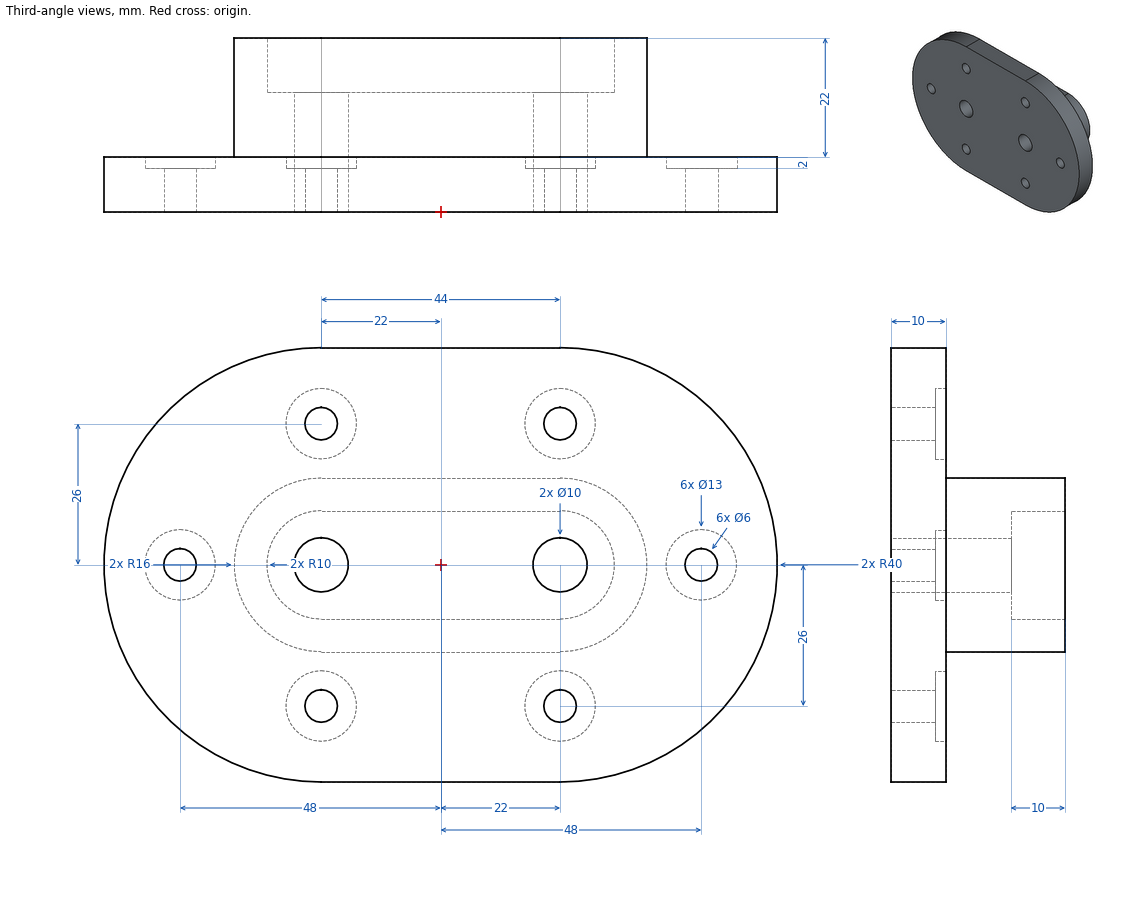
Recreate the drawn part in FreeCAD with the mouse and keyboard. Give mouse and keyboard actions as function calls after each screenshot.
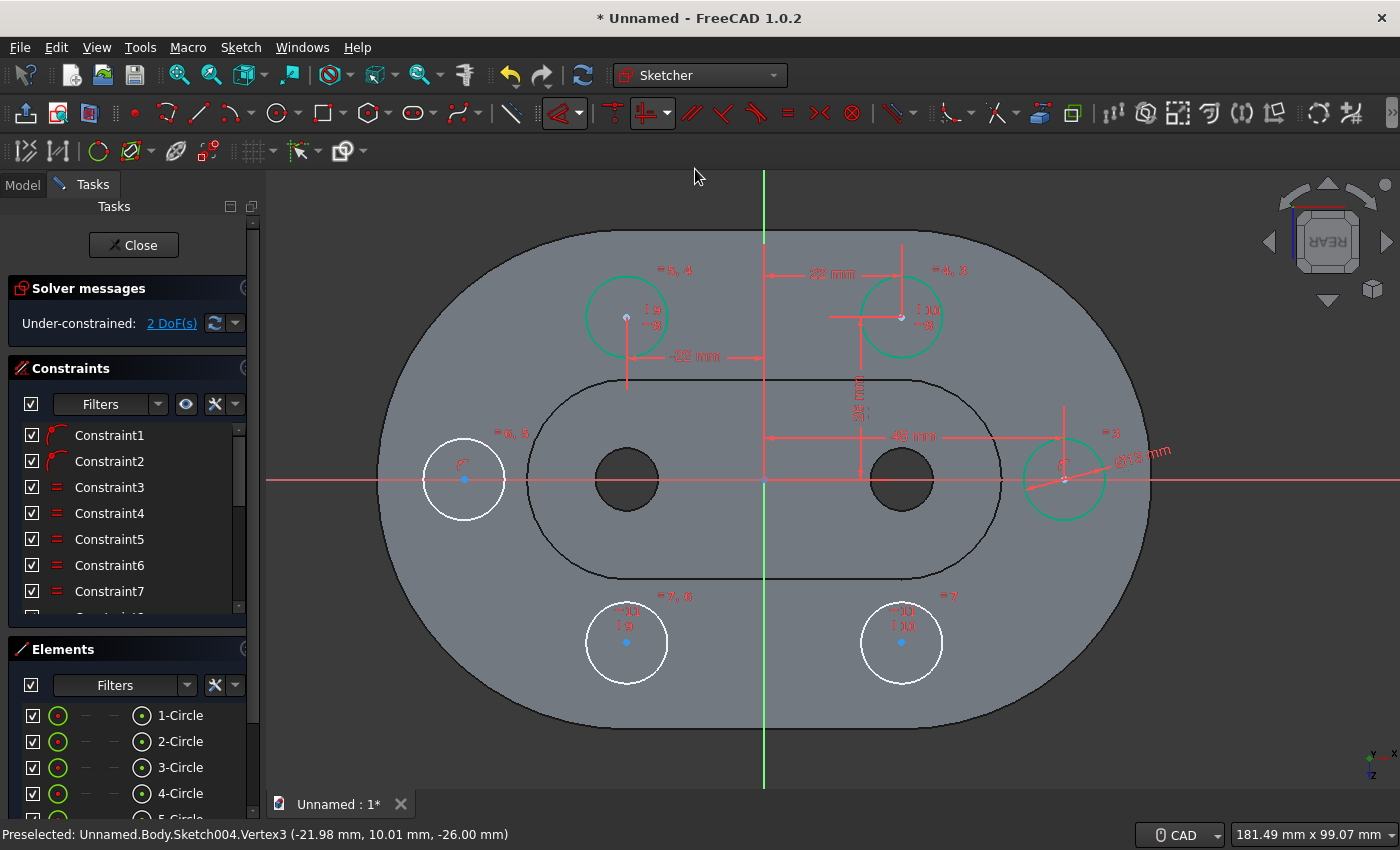
click(464, 479)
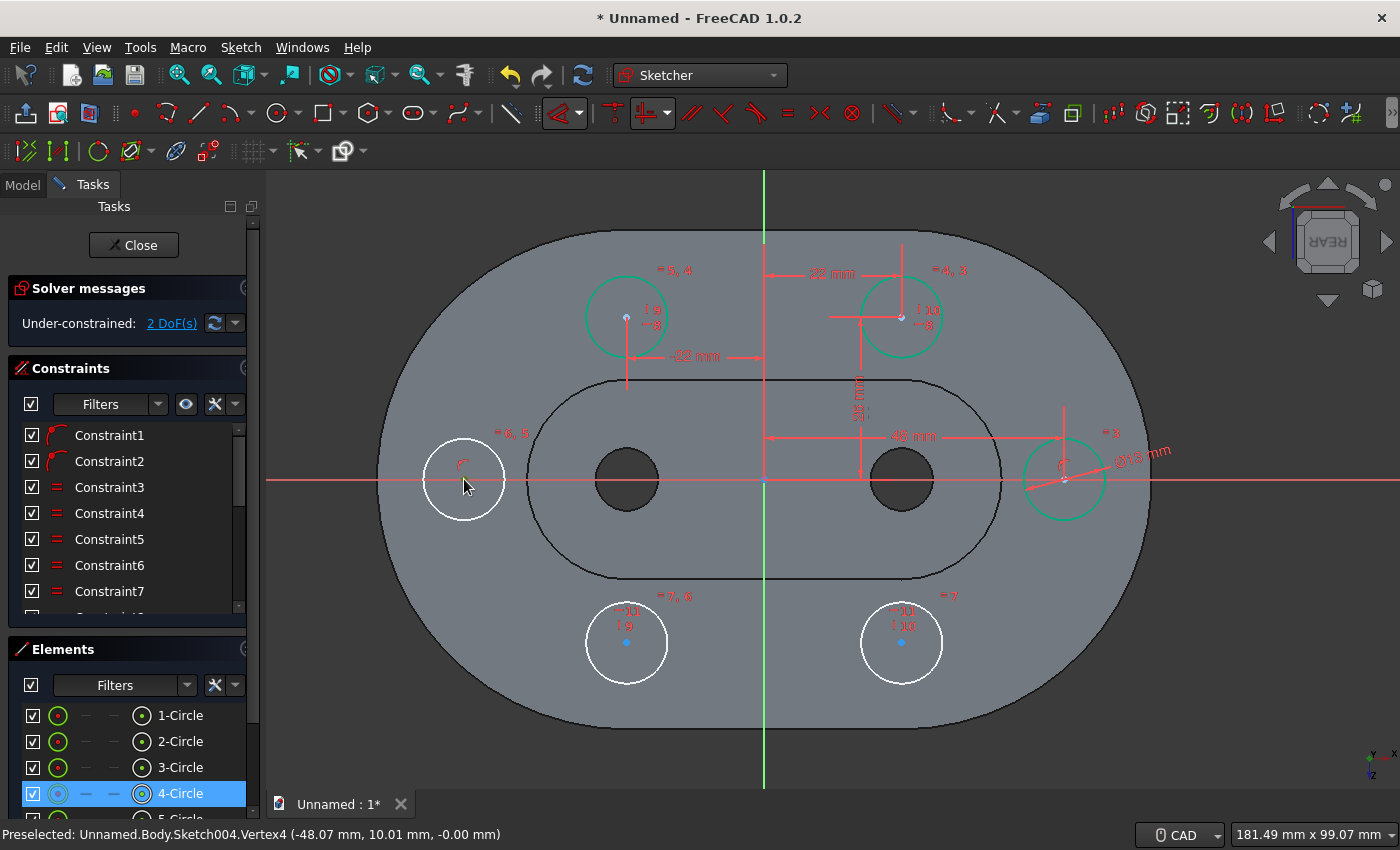
click(582, 114)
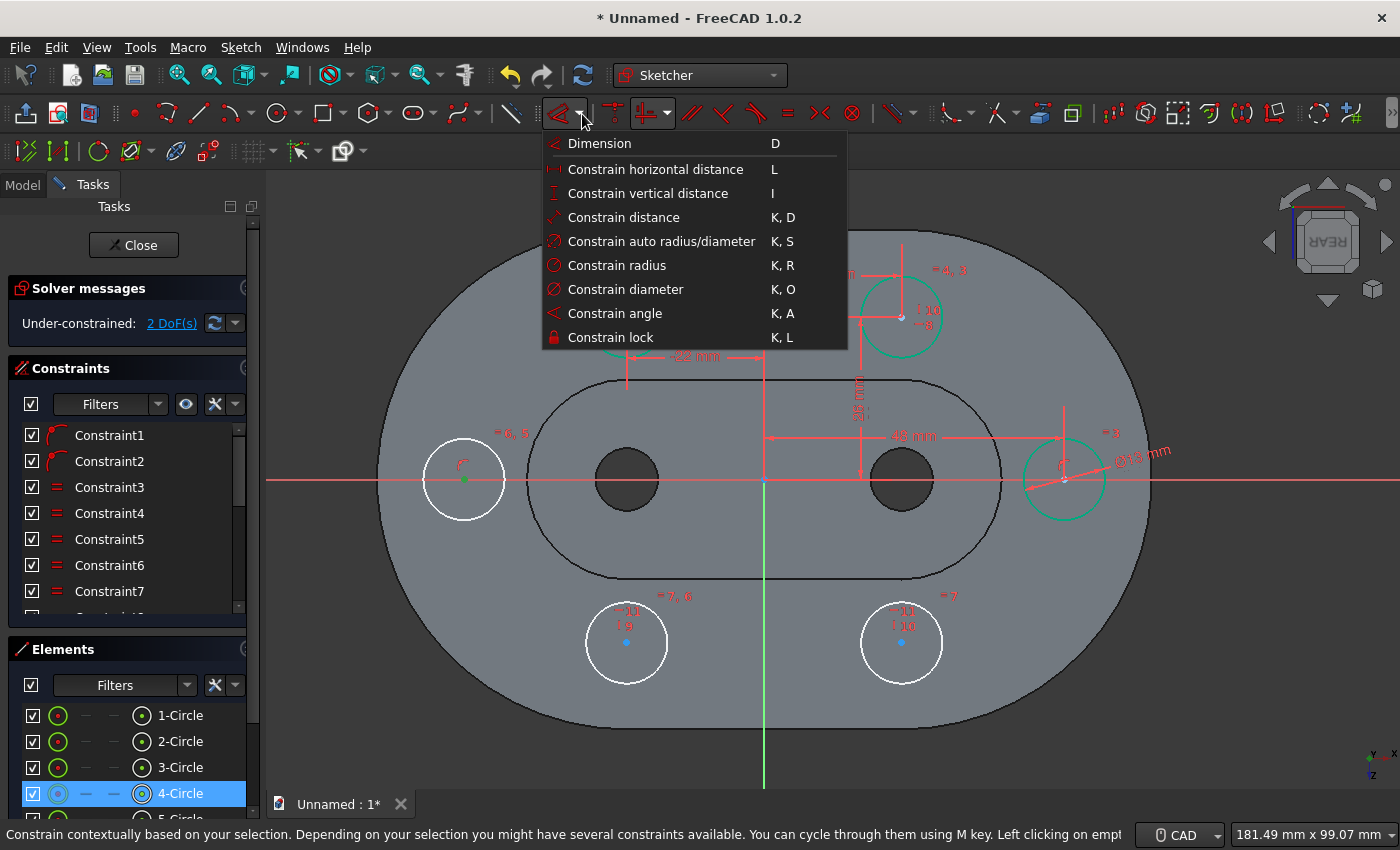
click(695, 169)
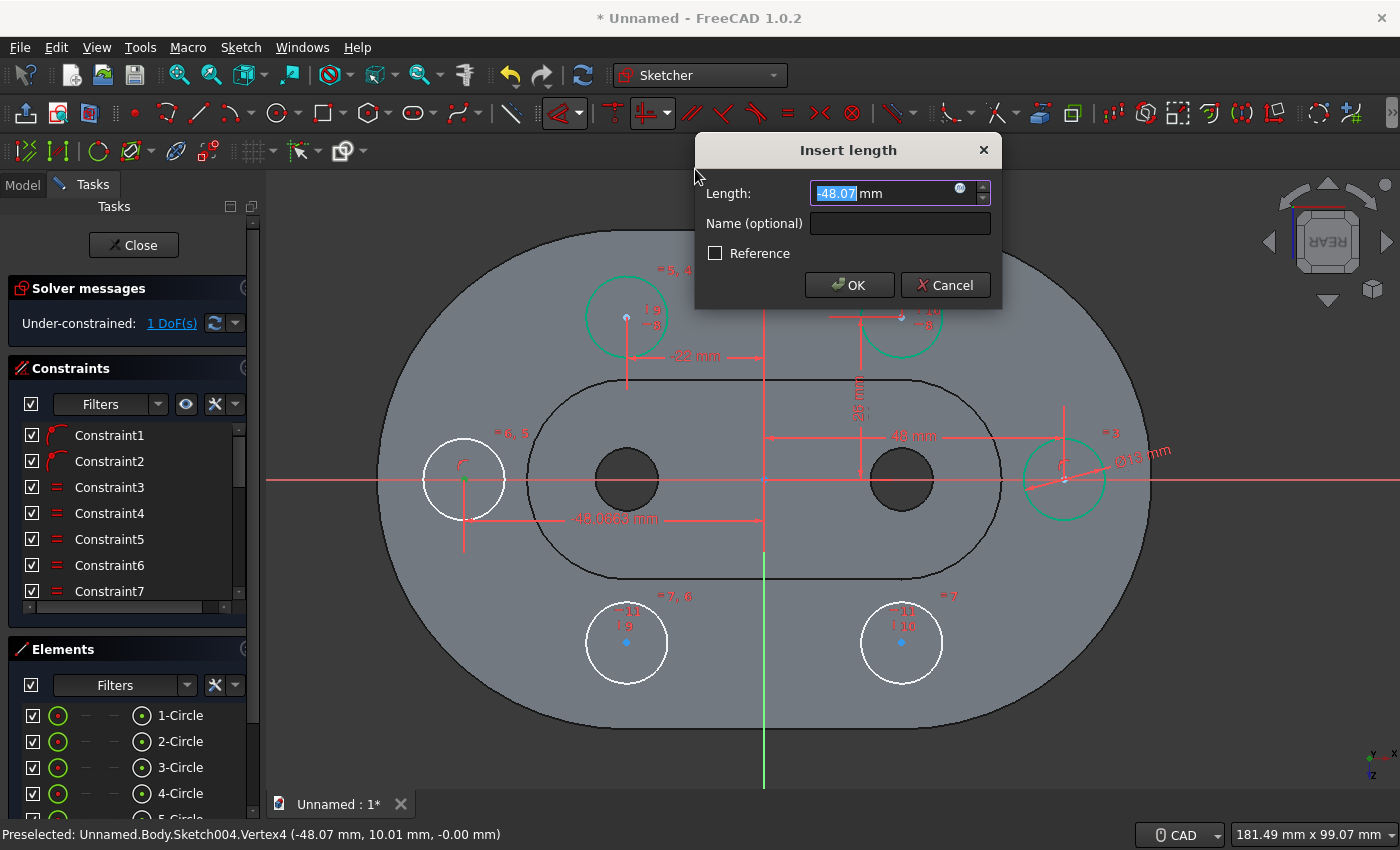
text(-48)
key(Return)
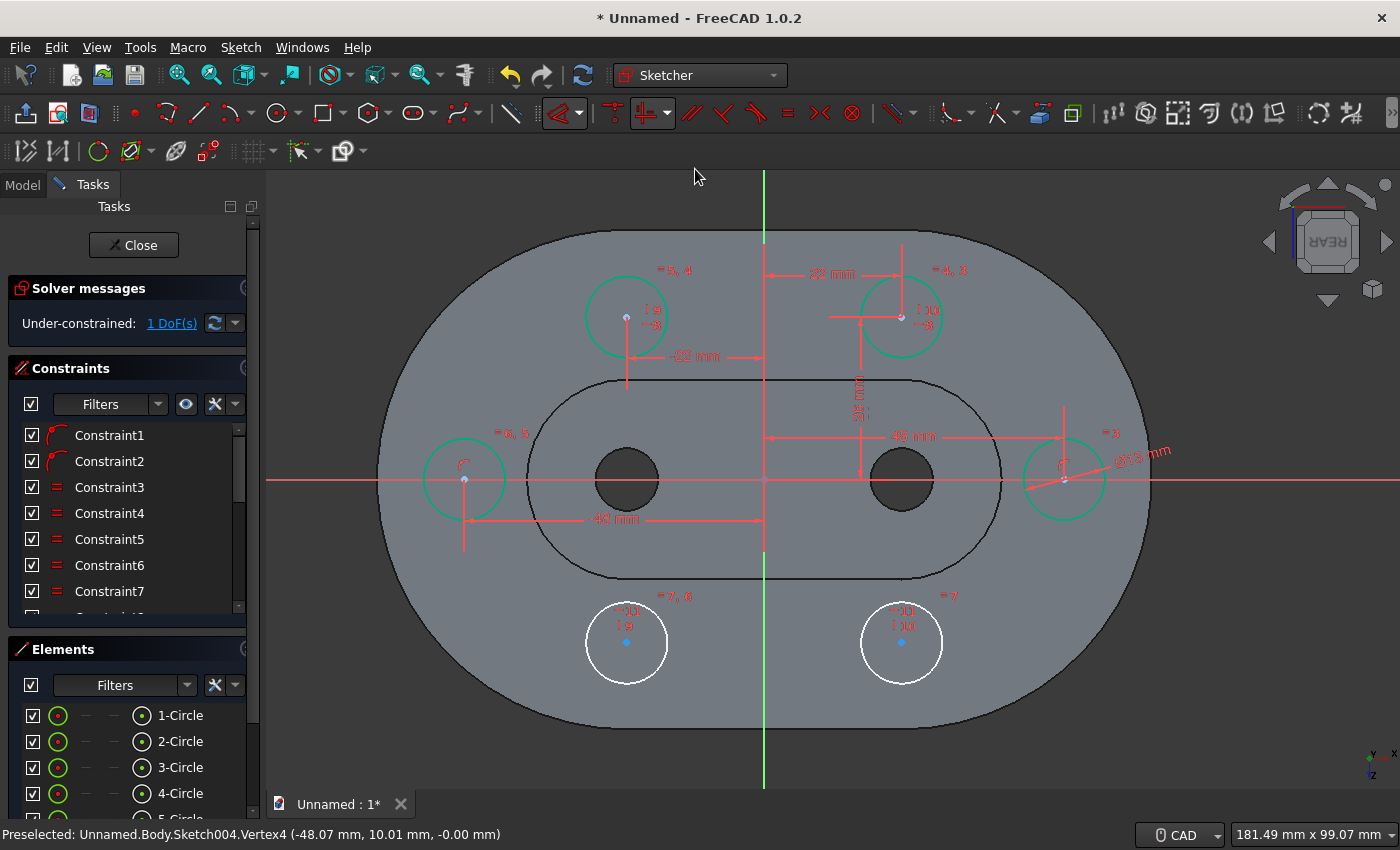
click(627, 643)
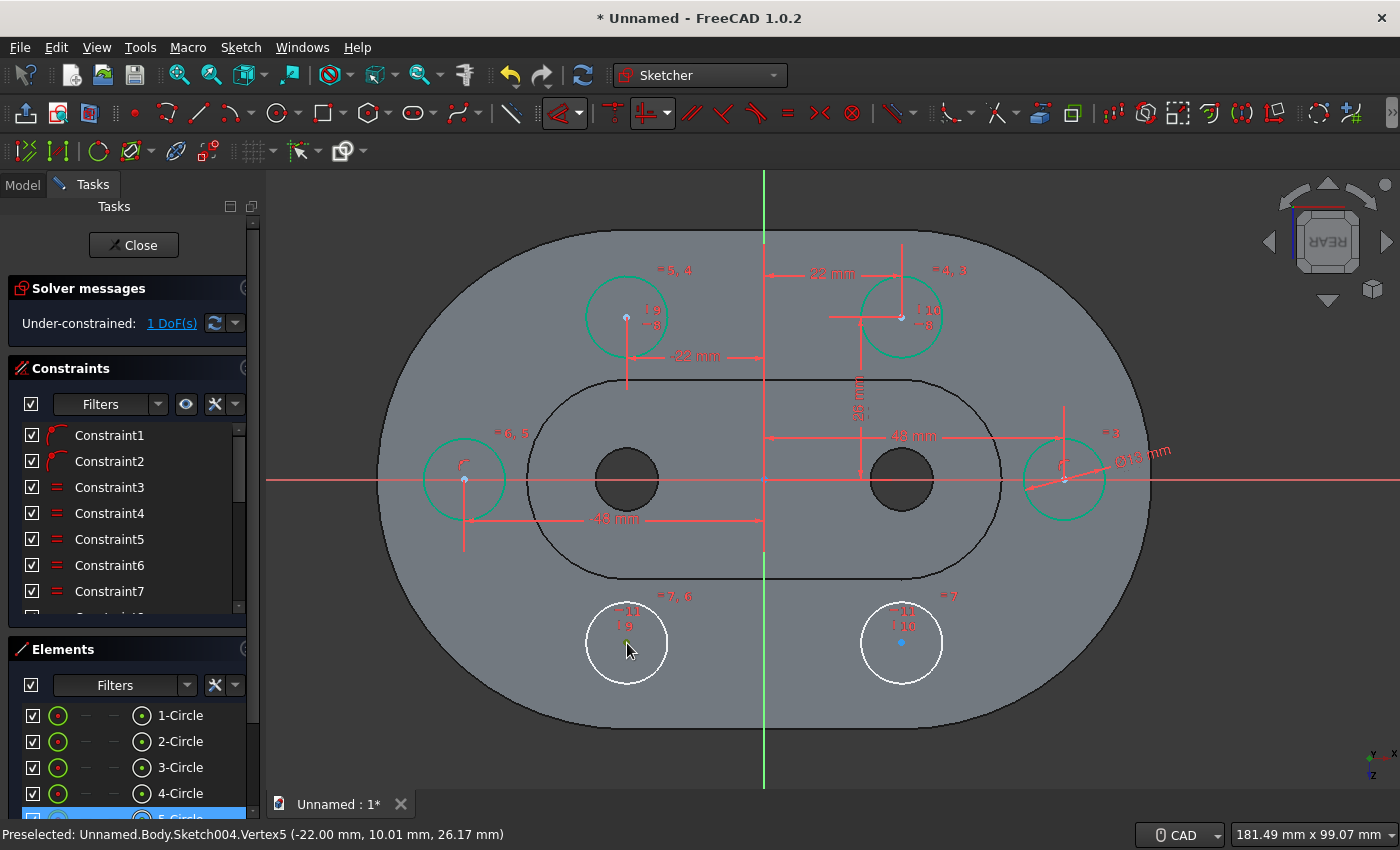
key(i)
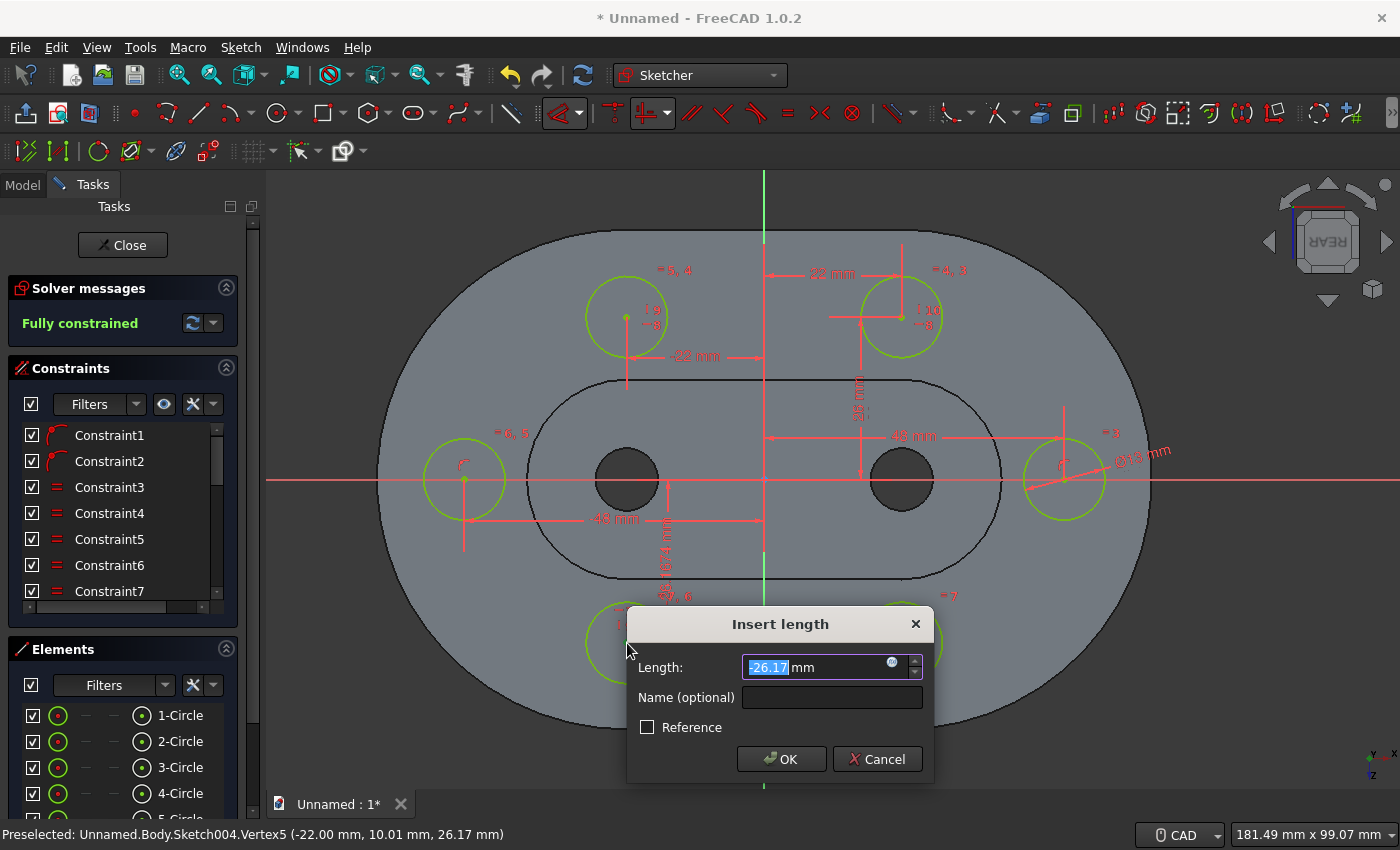
text(-26)
key(Return)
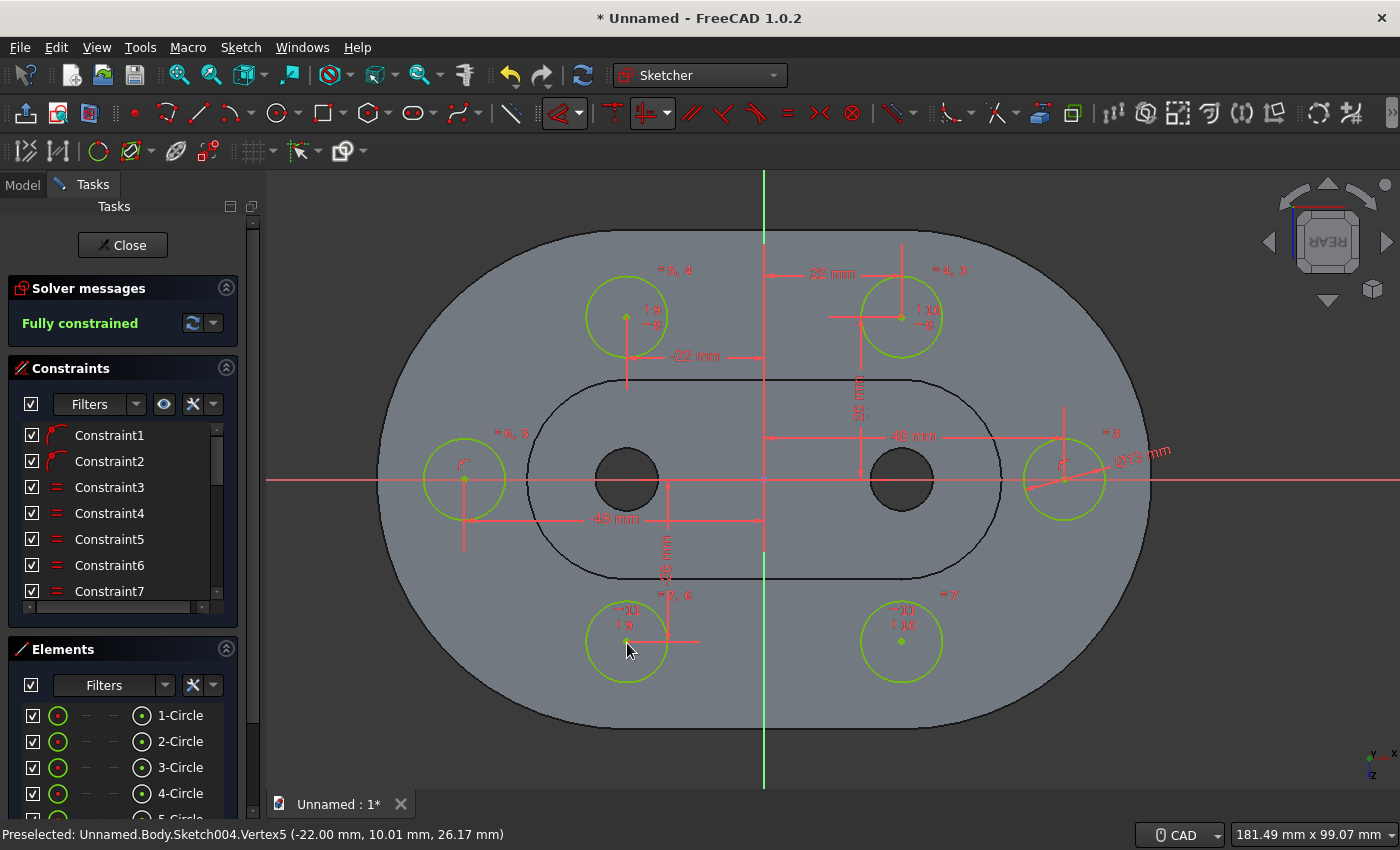
click(123, 245)